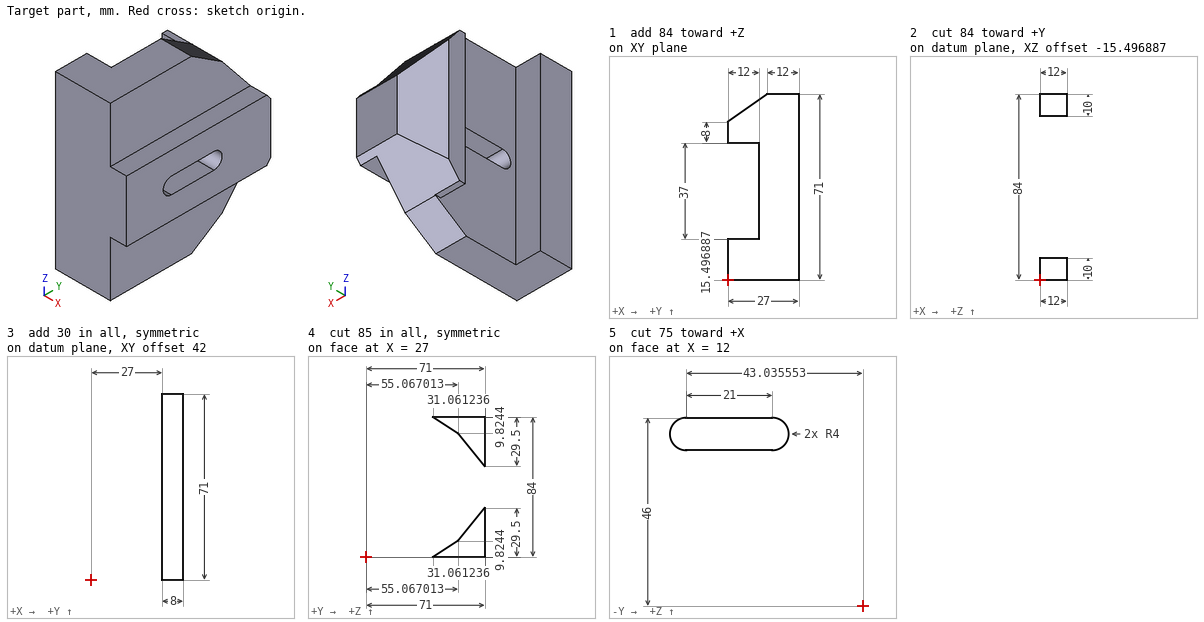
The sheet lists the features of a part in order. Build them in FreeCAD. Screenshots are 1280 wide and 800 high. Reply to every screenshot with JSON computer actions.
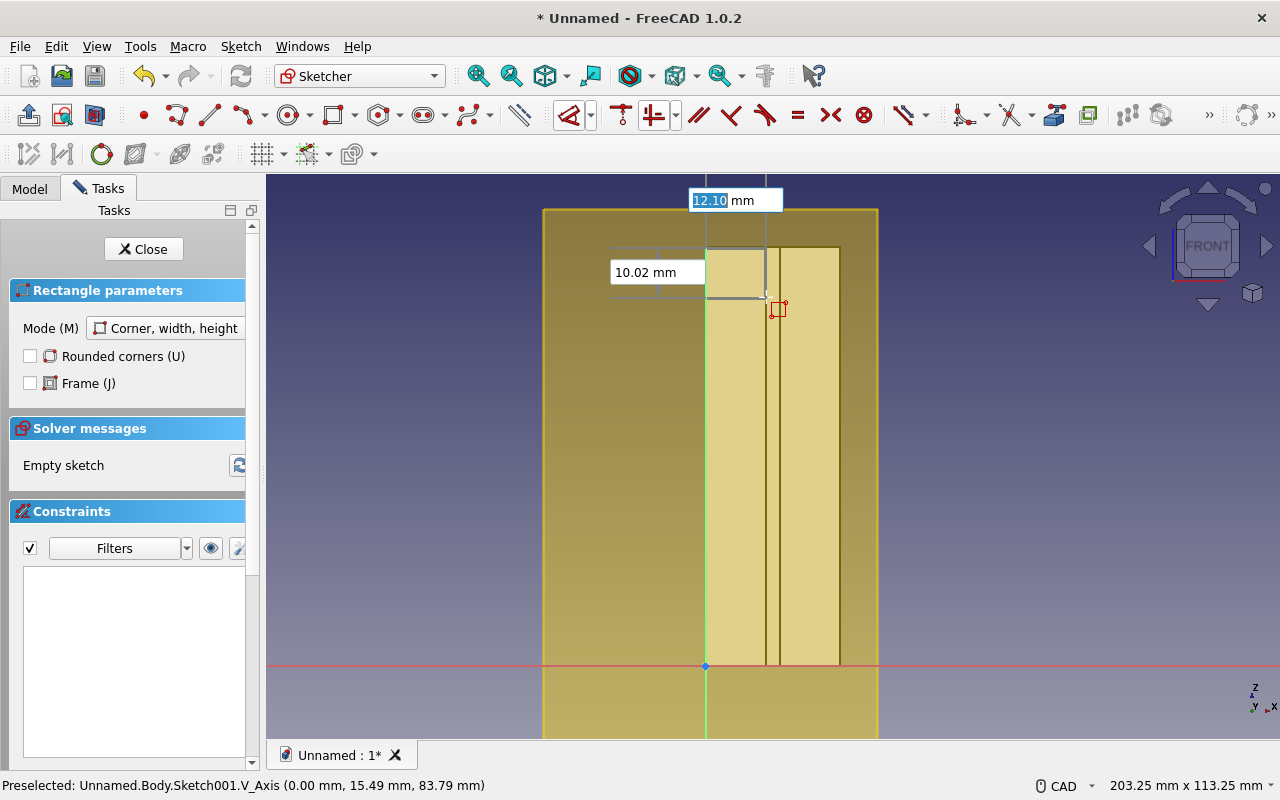
{"action": "type", "text": "12"}
{"action": "key", "text": "Tab"}
{"action": "type", "text": "10"}
{"action": "key", "text": "Return"}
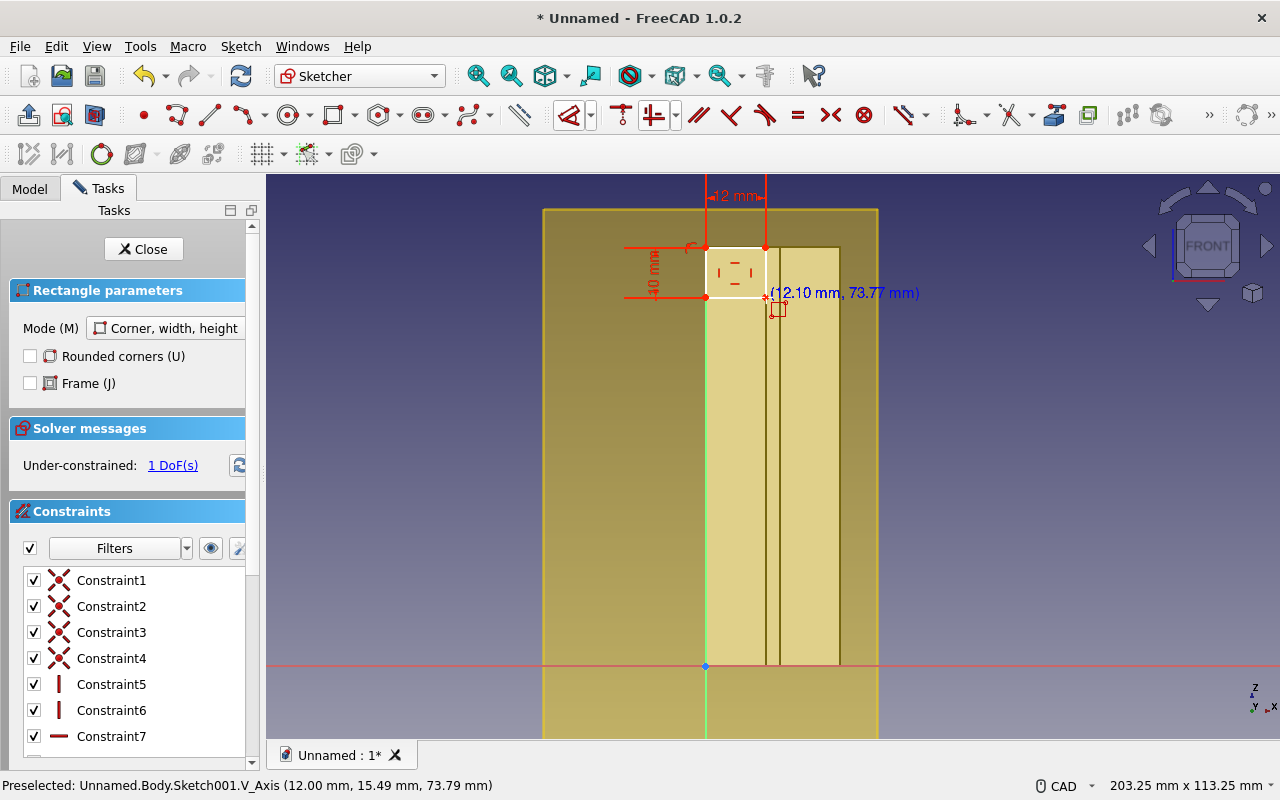
{"action": "left_click", "coordinate": [706, 666]}
{"action": "mouse_move", "coordinate": [766, 616]}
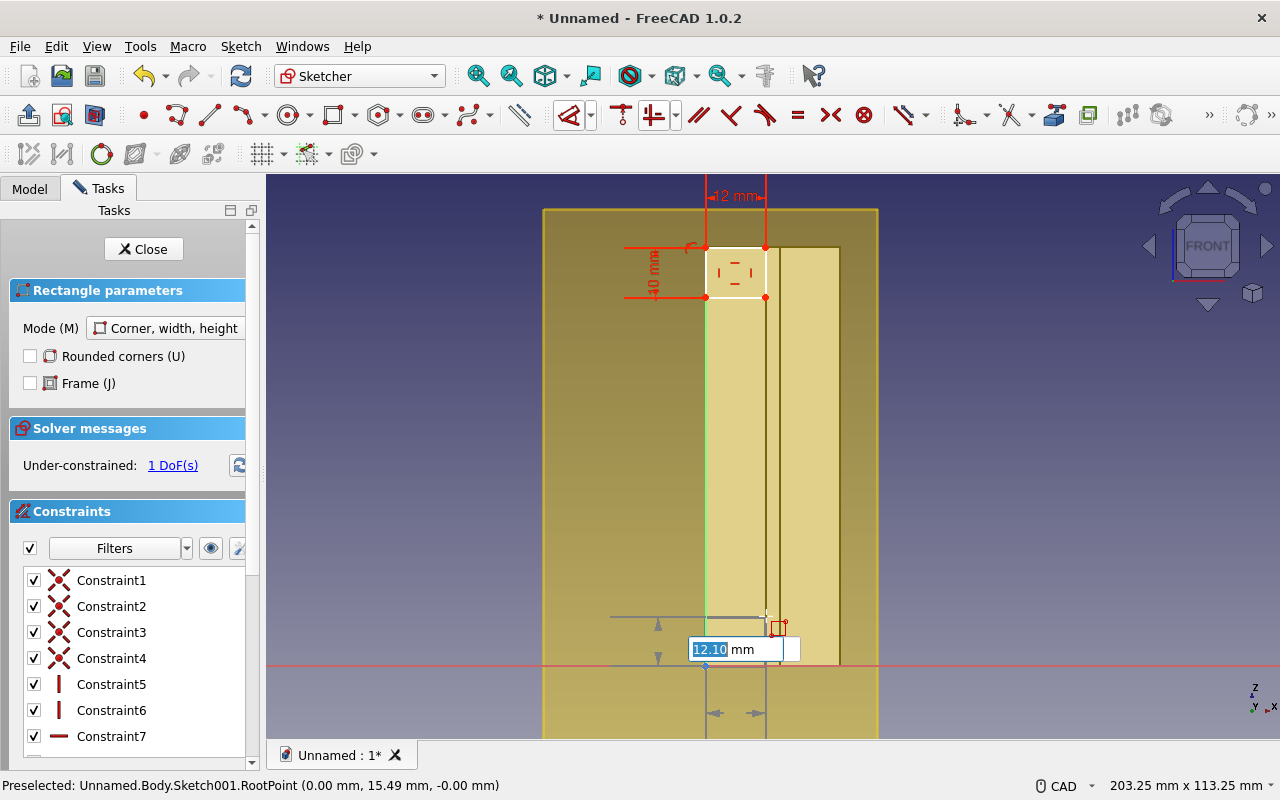
{"action": "type", "text": "12"}
{"action": "key", "text": "Tab"}
{"action": "type", "text": "10"}
{"action": "key", "text": "Return"}
{"action": "key", "text": "Escape"}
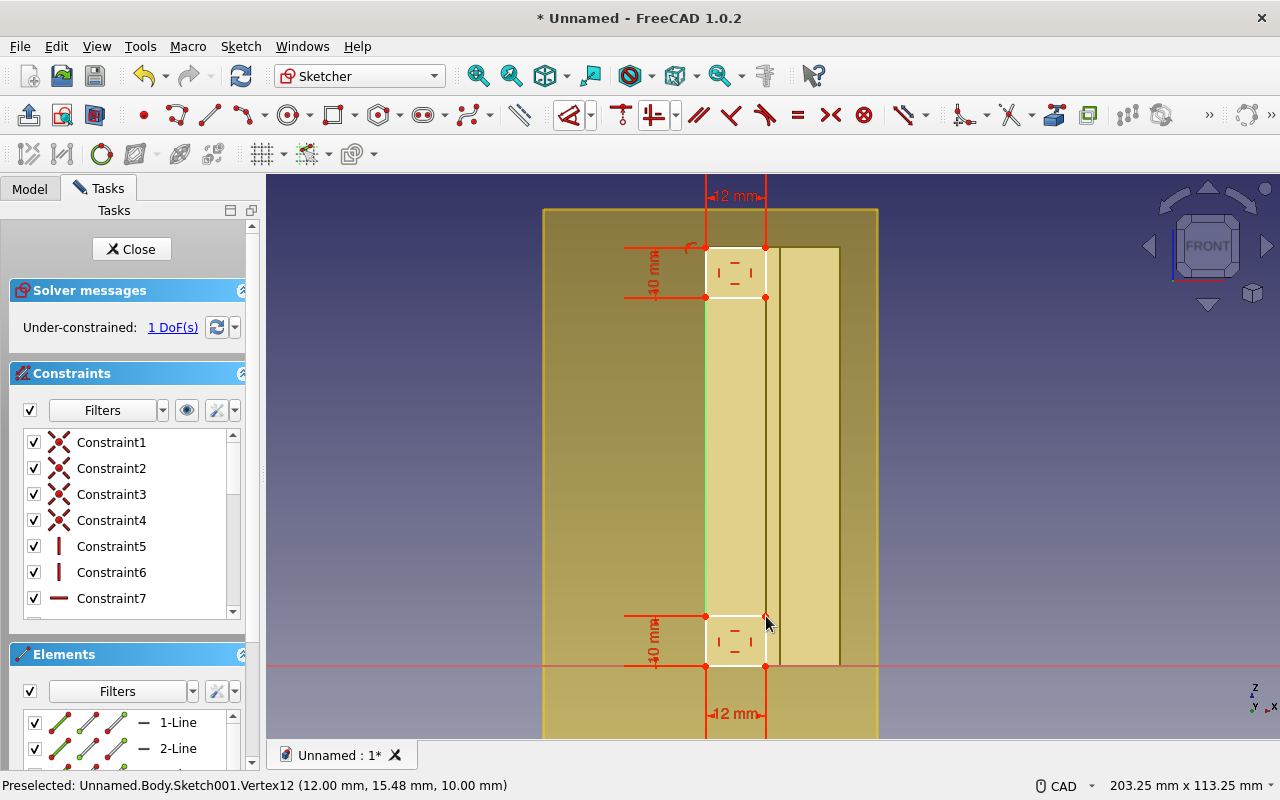
{"action": "left_click", "coordinate": [706, 248]}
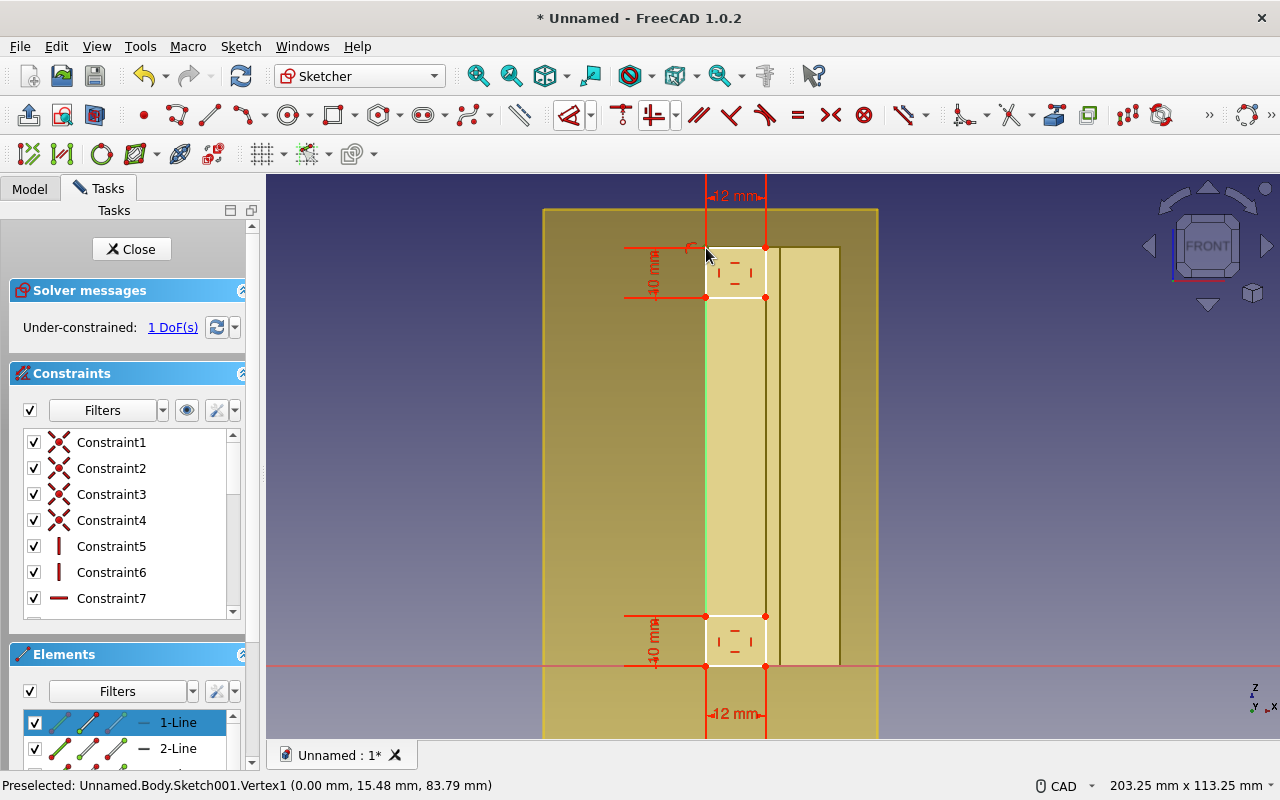
{"action": "key", "text": "i"}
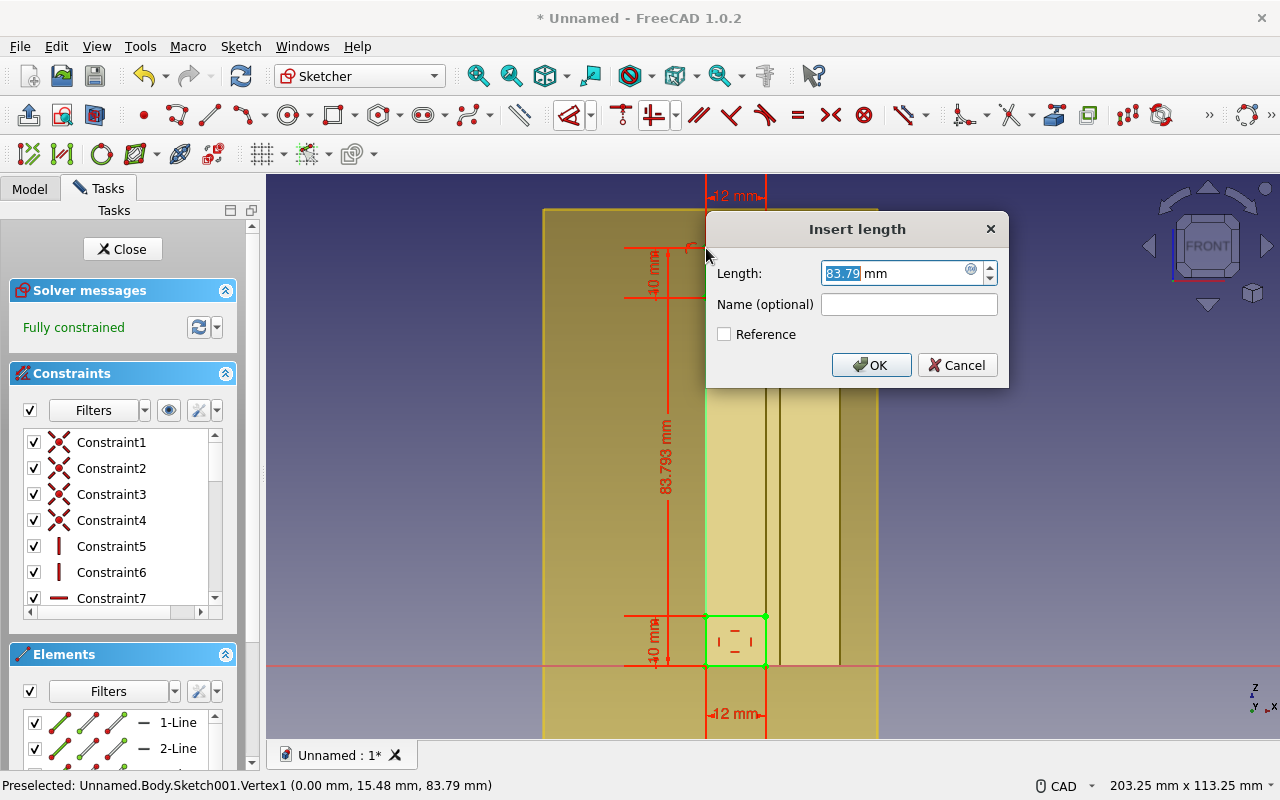
{"action": "type", "text": "84"}
{"action": "key", "text": "Return"}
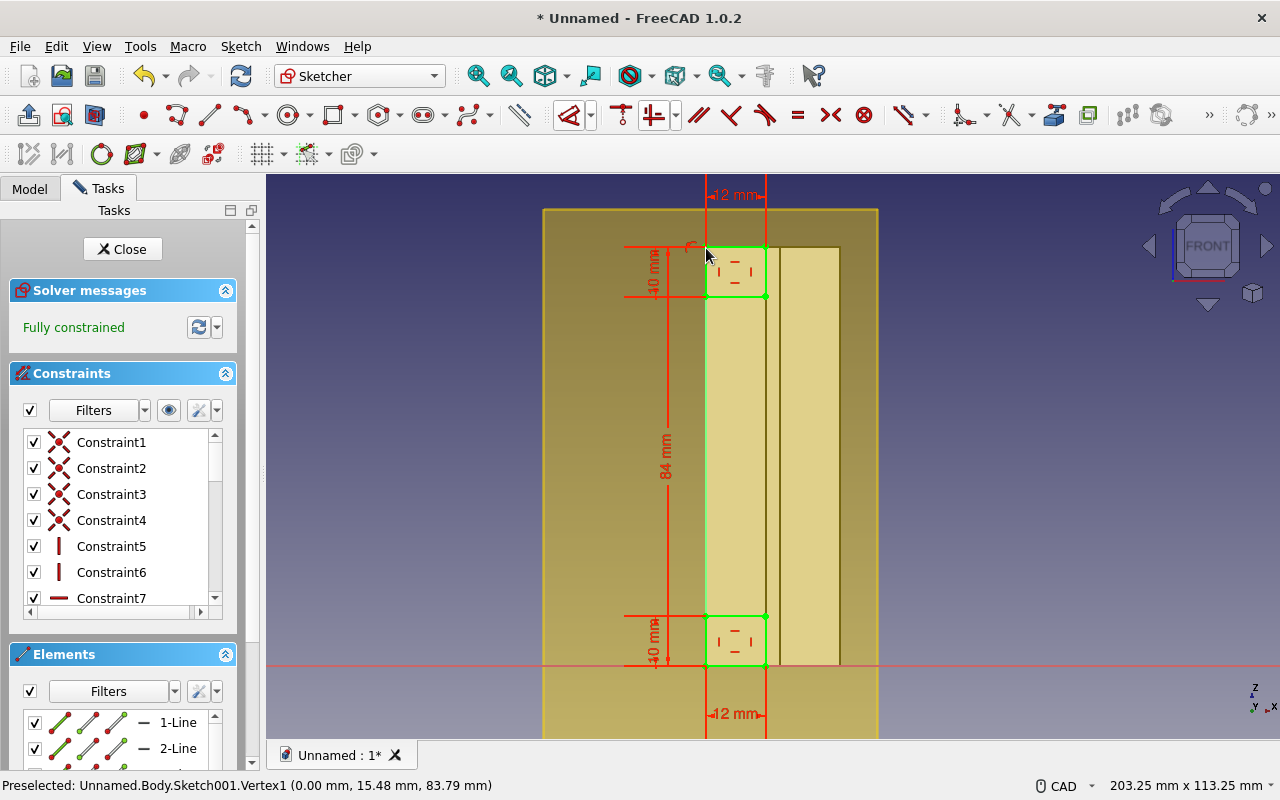
{"action": "left_click", "coordinate": [123, 249]}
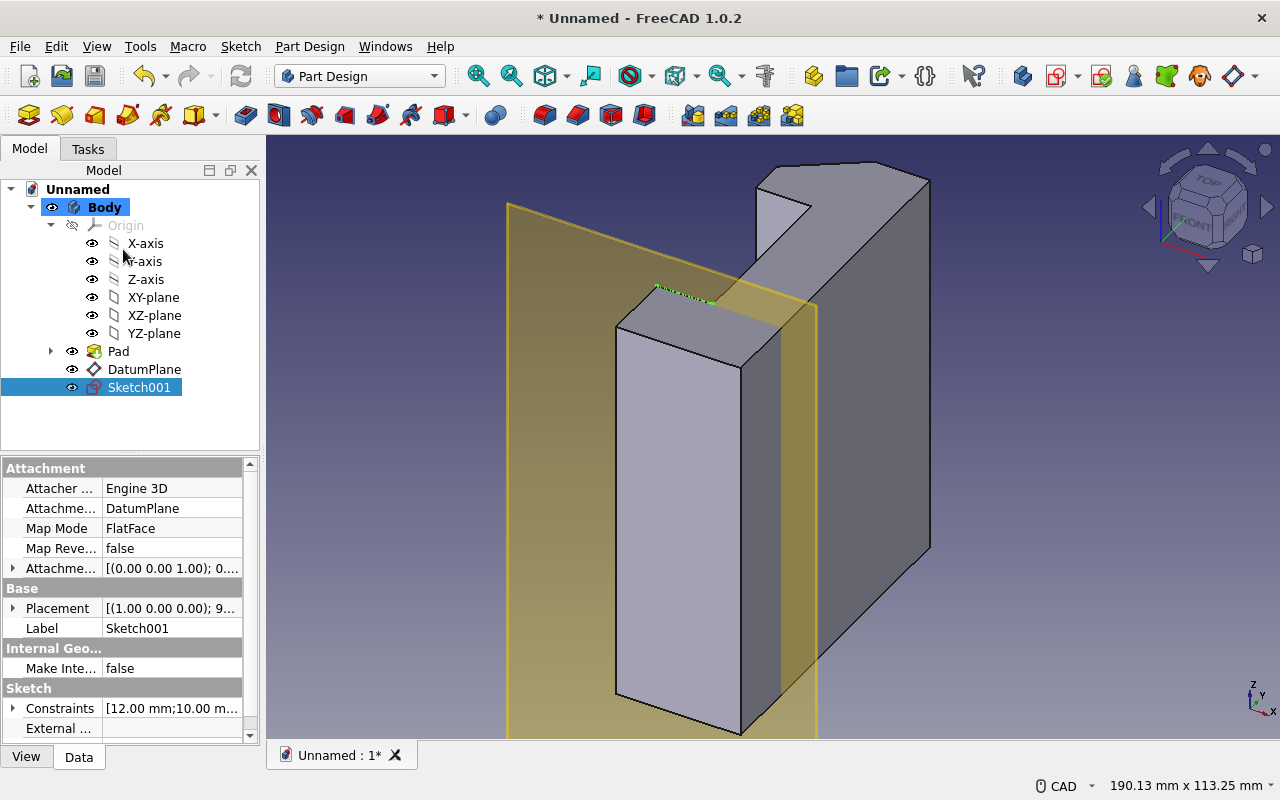
{"action": "left_click", "coordinate": [246, 116]}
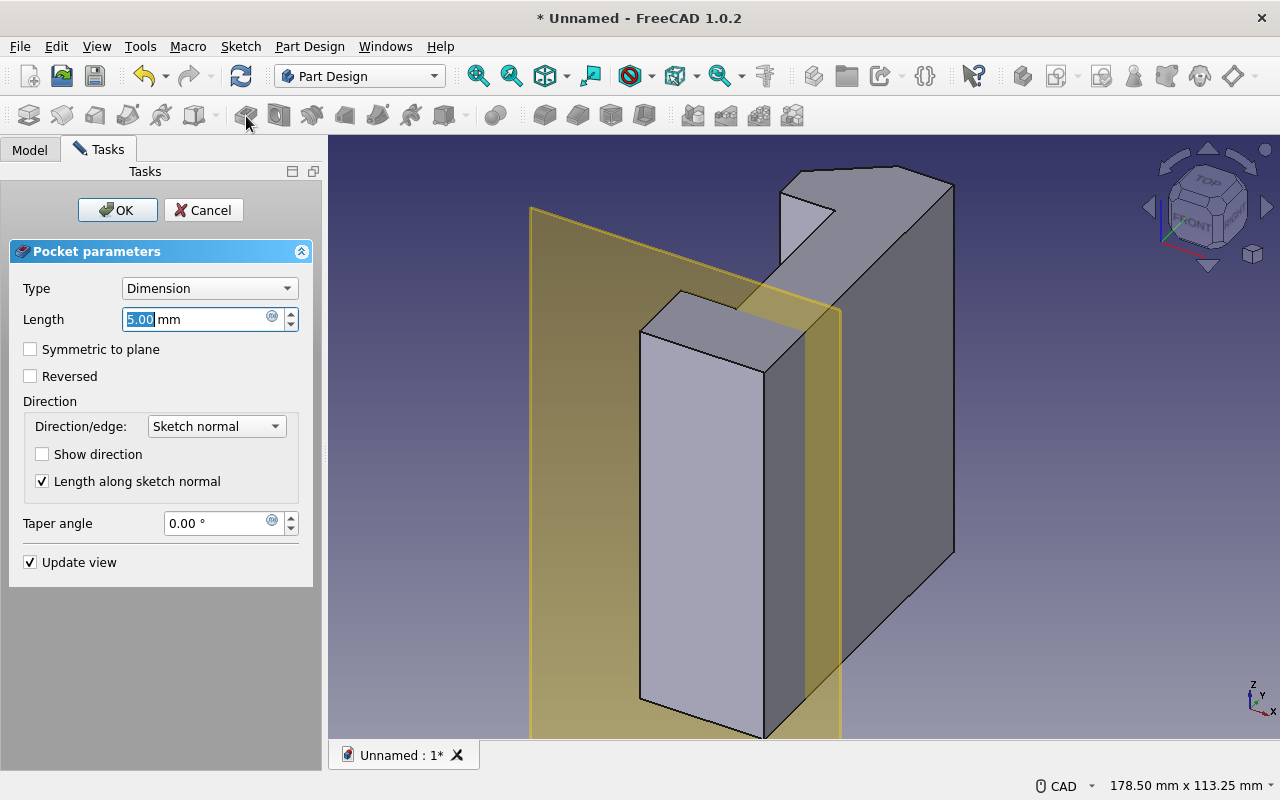
{"action": "type", "text": "84"}
{"action": "key", "text": "Tab"}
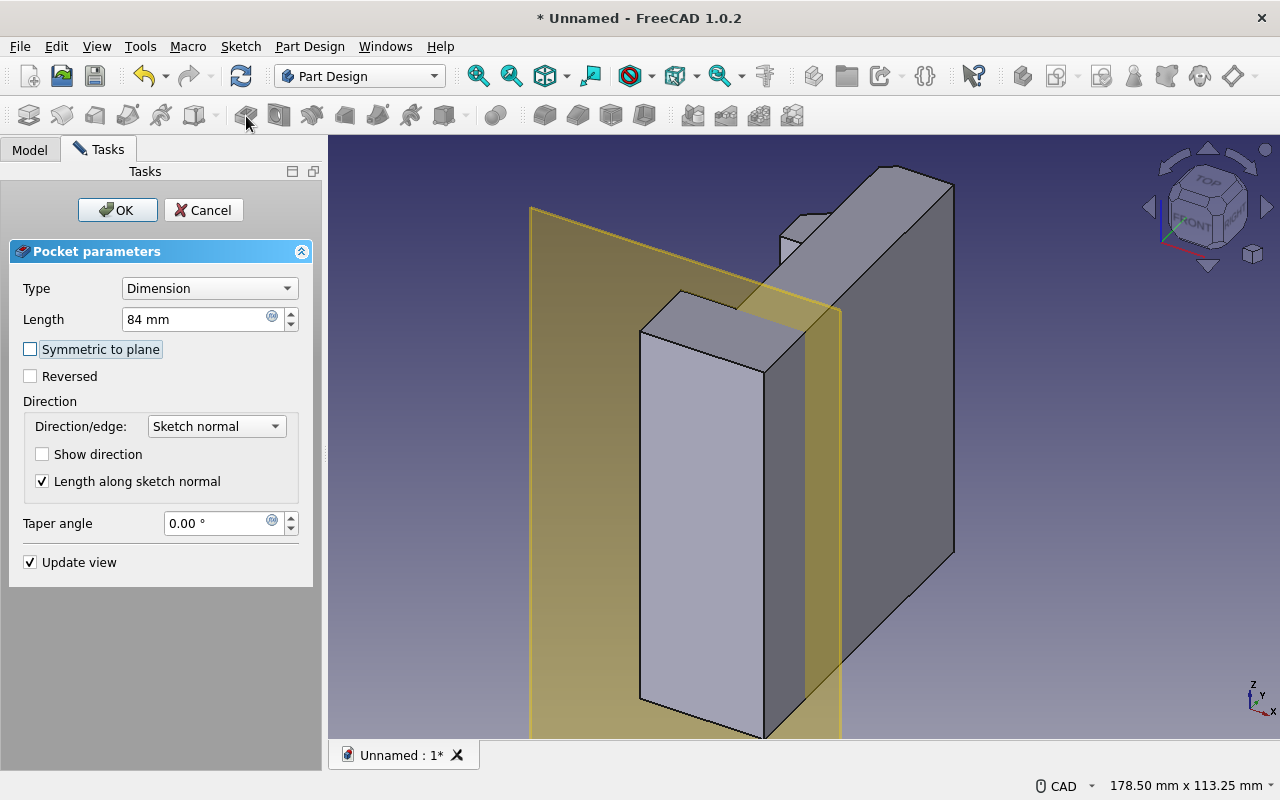
{"action": "left_click", "coordinate": [118, 210]}